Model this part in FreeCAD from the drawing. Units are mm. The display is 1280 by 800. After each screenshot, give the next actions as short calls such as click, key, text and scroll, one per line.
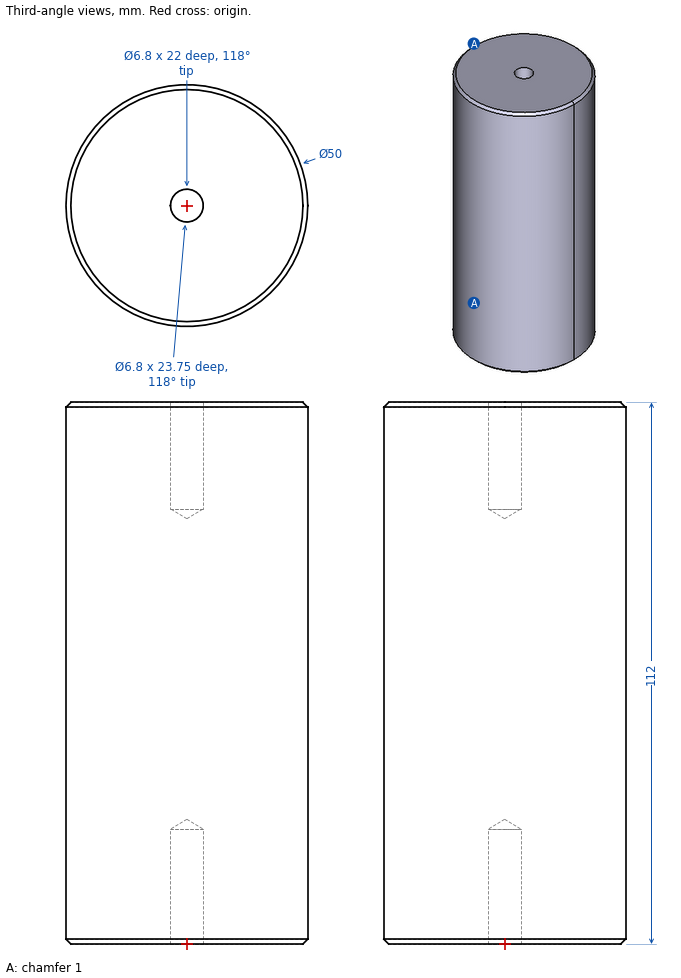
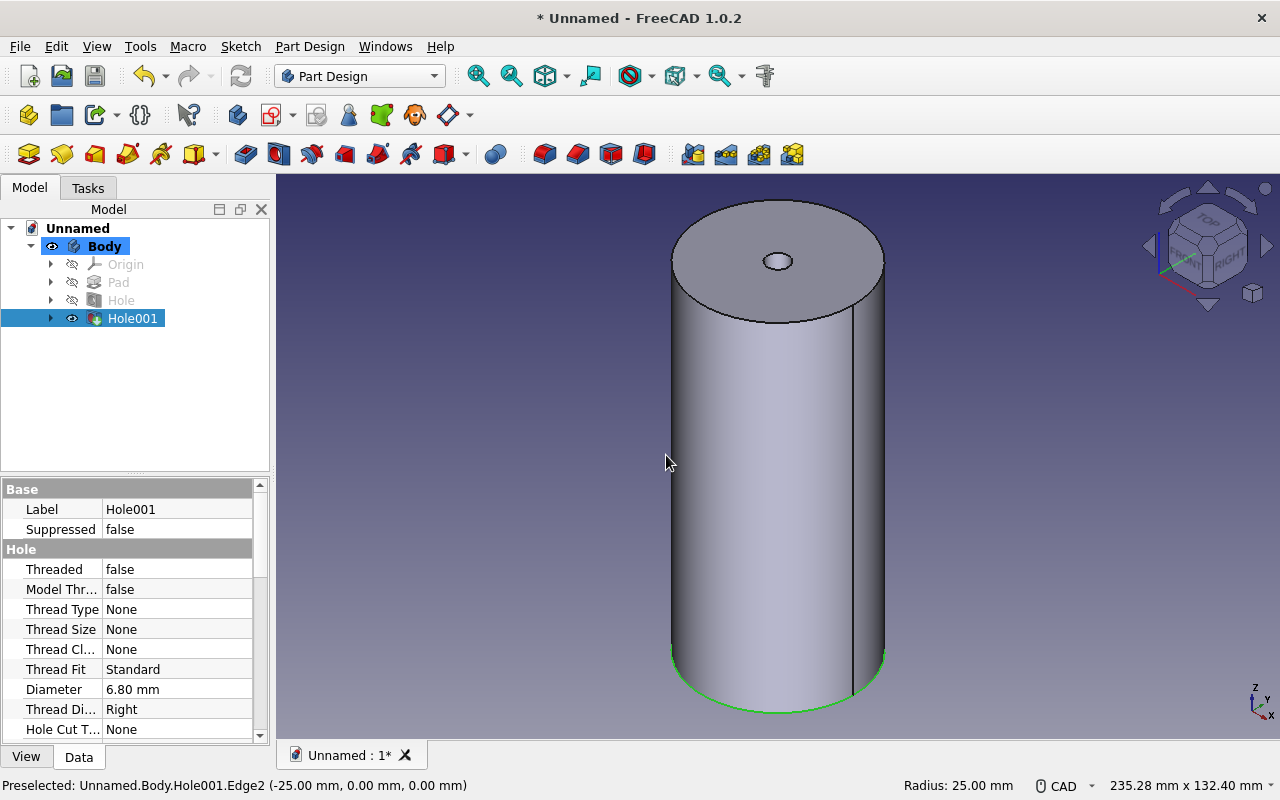
click(683, 288, ctrl)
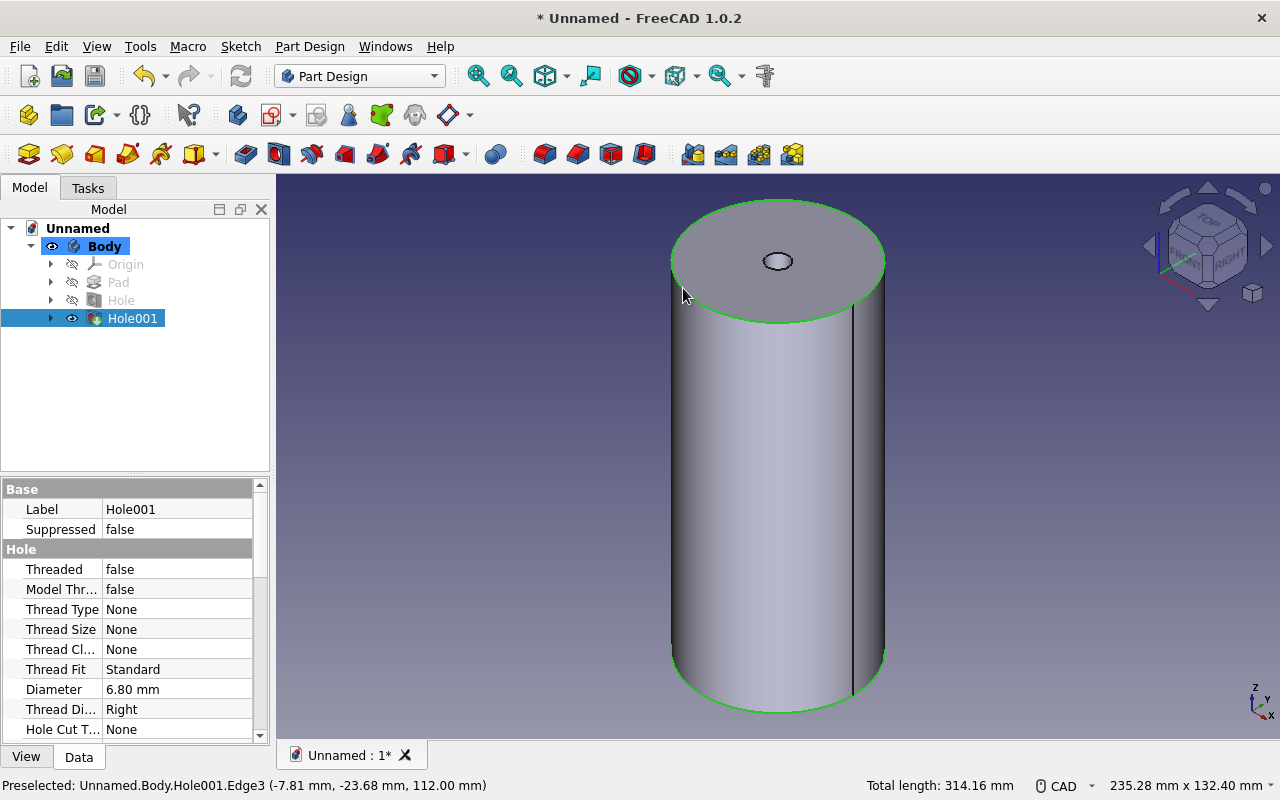
click(578, 154)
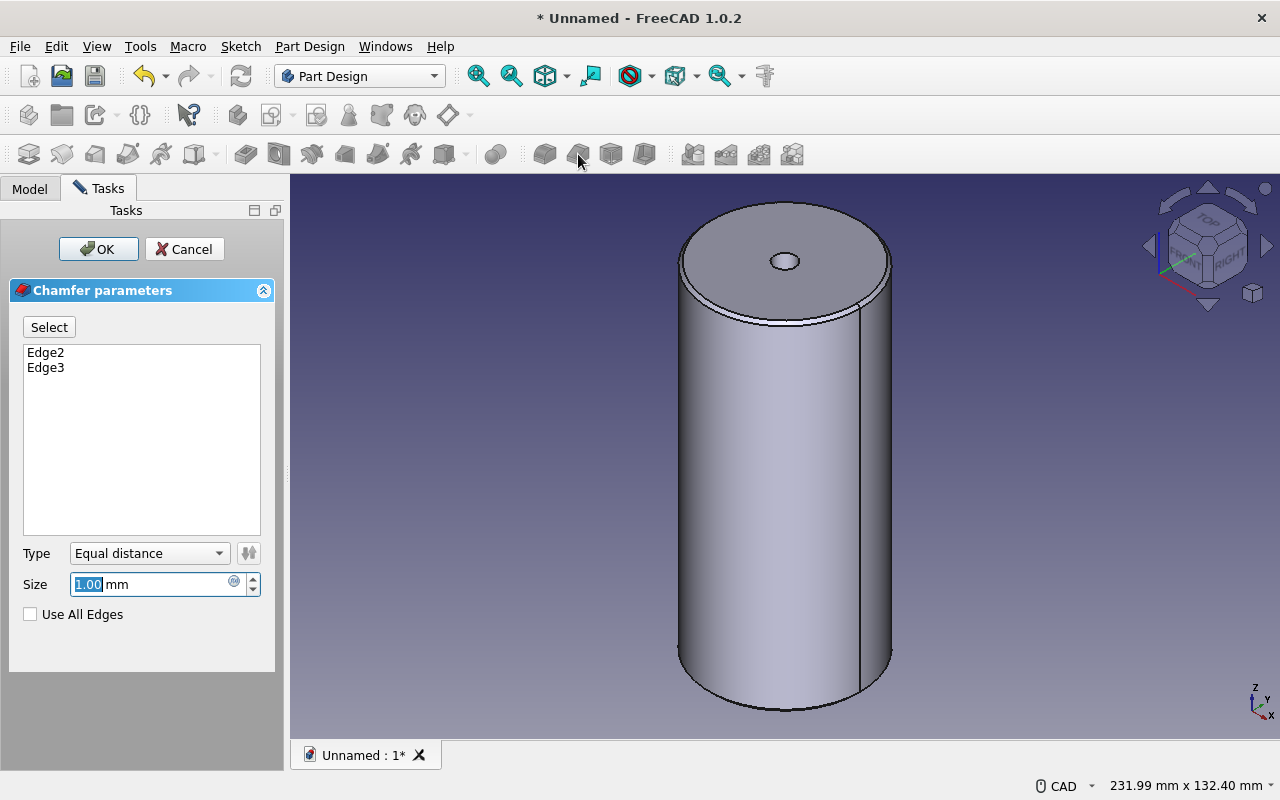
text(1)
key(Tab)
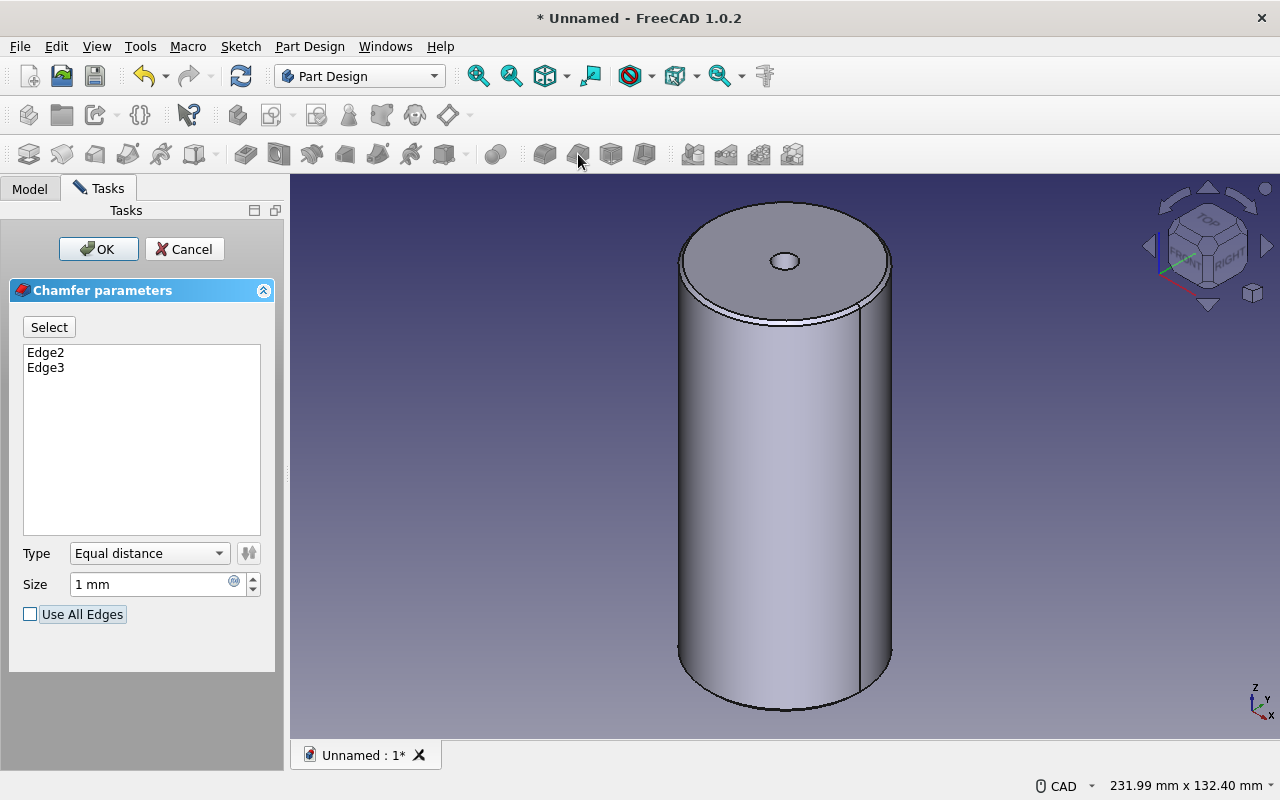
click(99, 249)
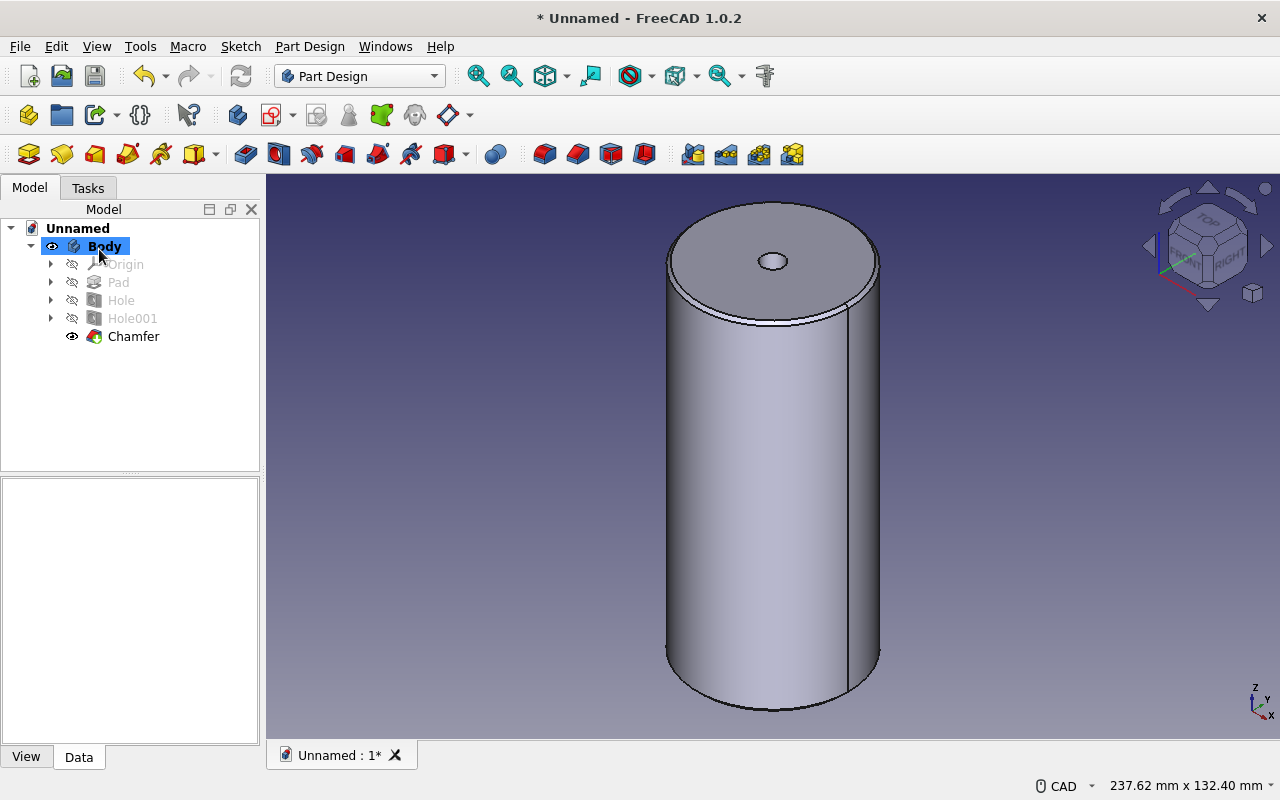
key(v)
key(f)